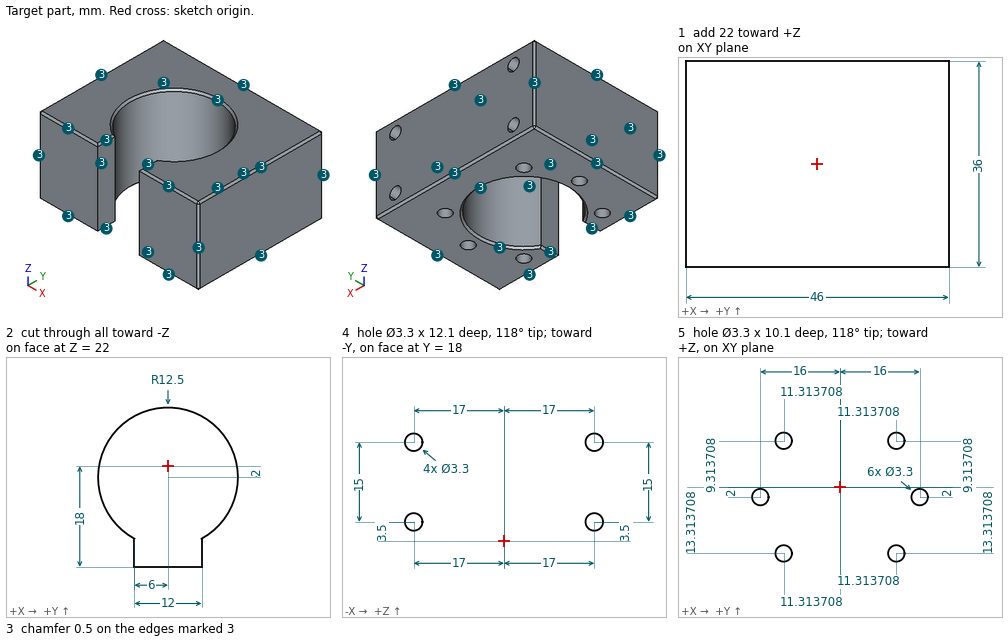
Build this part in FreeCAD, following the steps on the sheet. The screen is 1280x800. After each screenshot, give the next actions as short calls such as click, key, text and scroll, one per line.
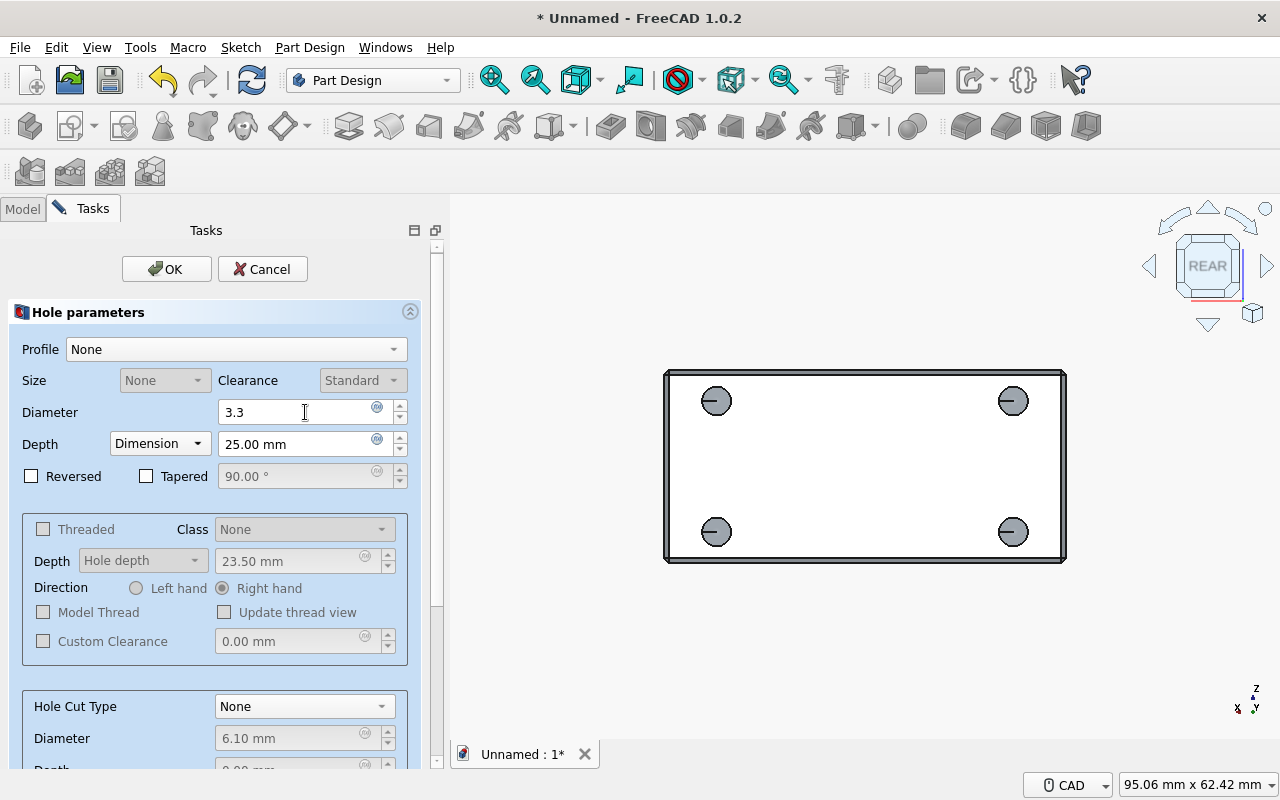
triple_click(305, 444)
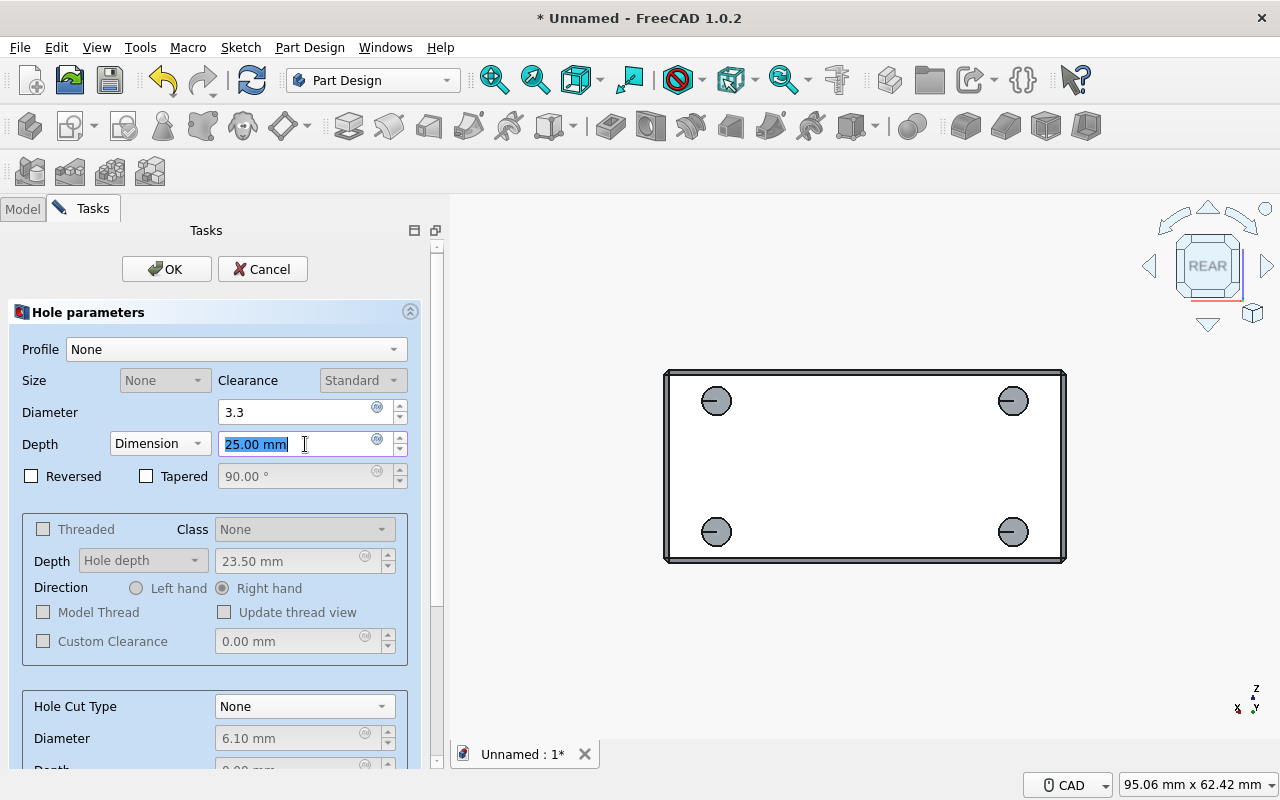
text(10.1)
key(Tab)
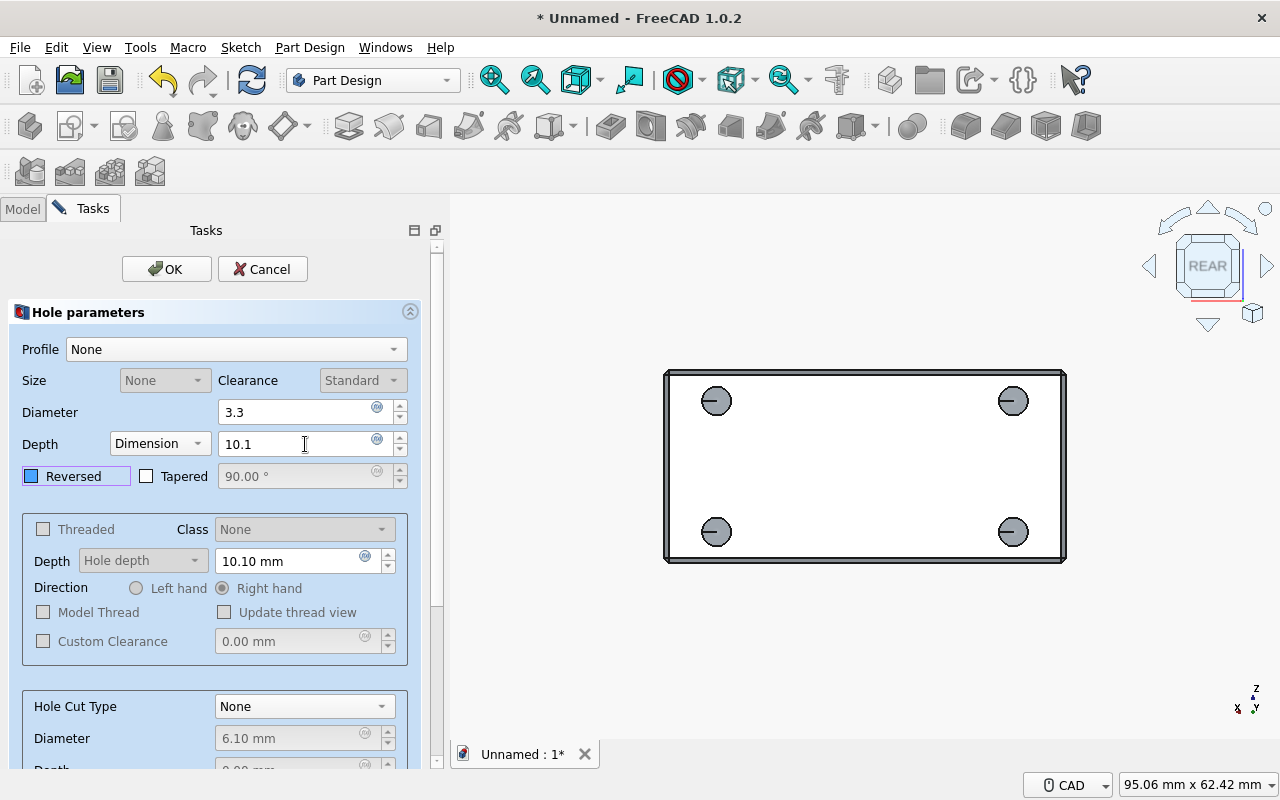
click(30, 476)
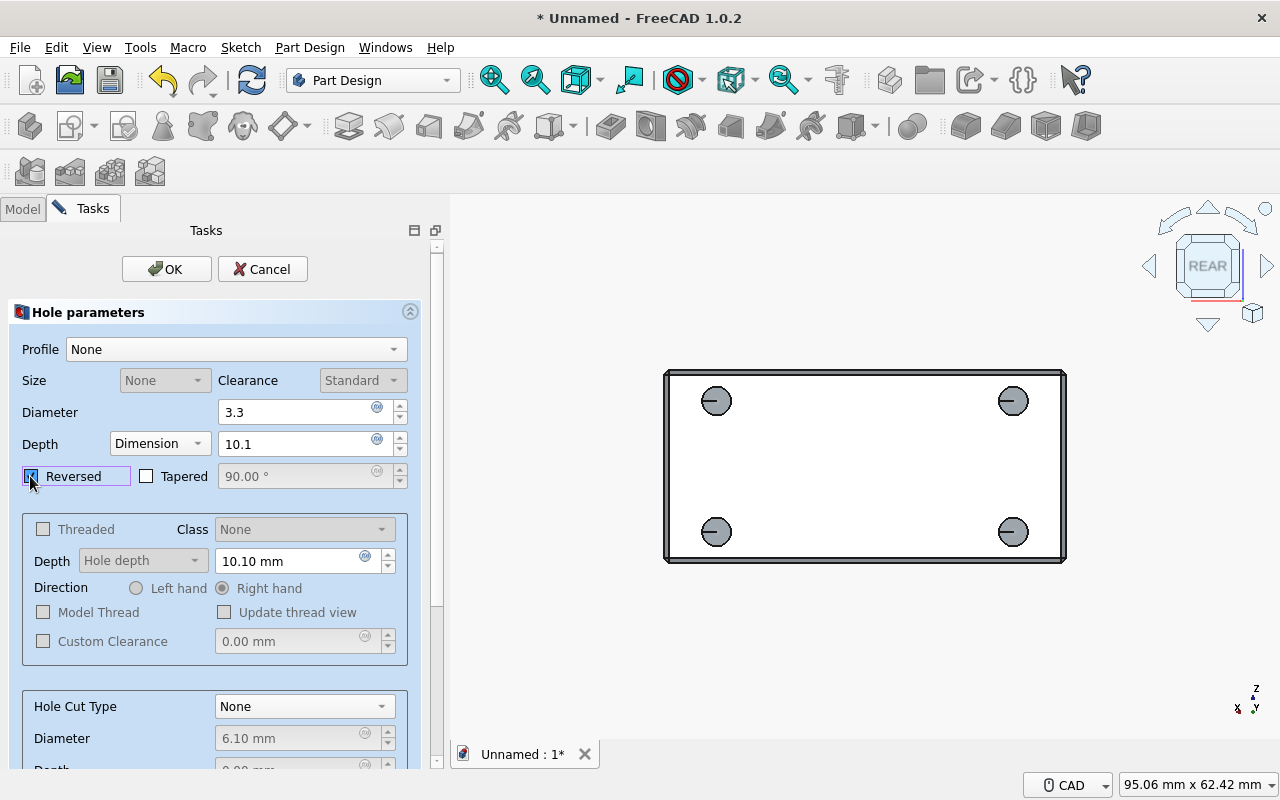
click(167, 269)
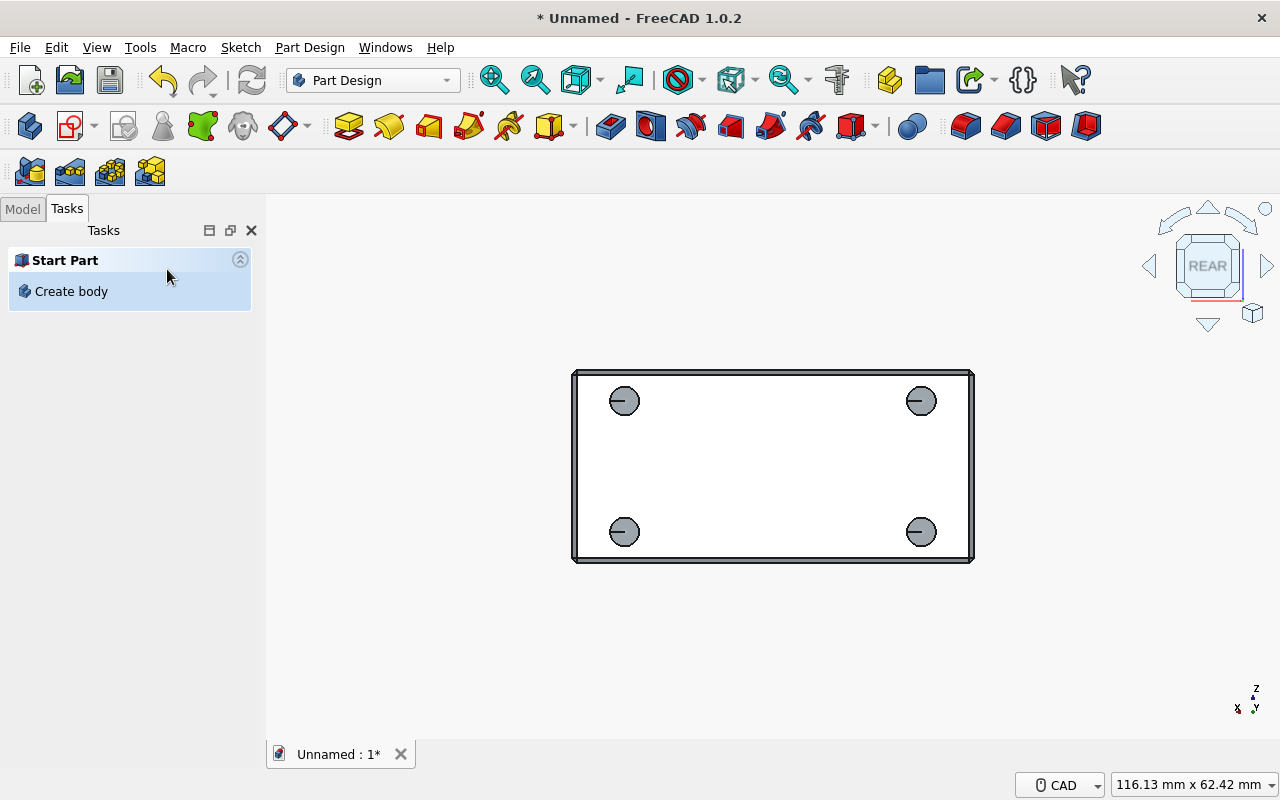
key(0)